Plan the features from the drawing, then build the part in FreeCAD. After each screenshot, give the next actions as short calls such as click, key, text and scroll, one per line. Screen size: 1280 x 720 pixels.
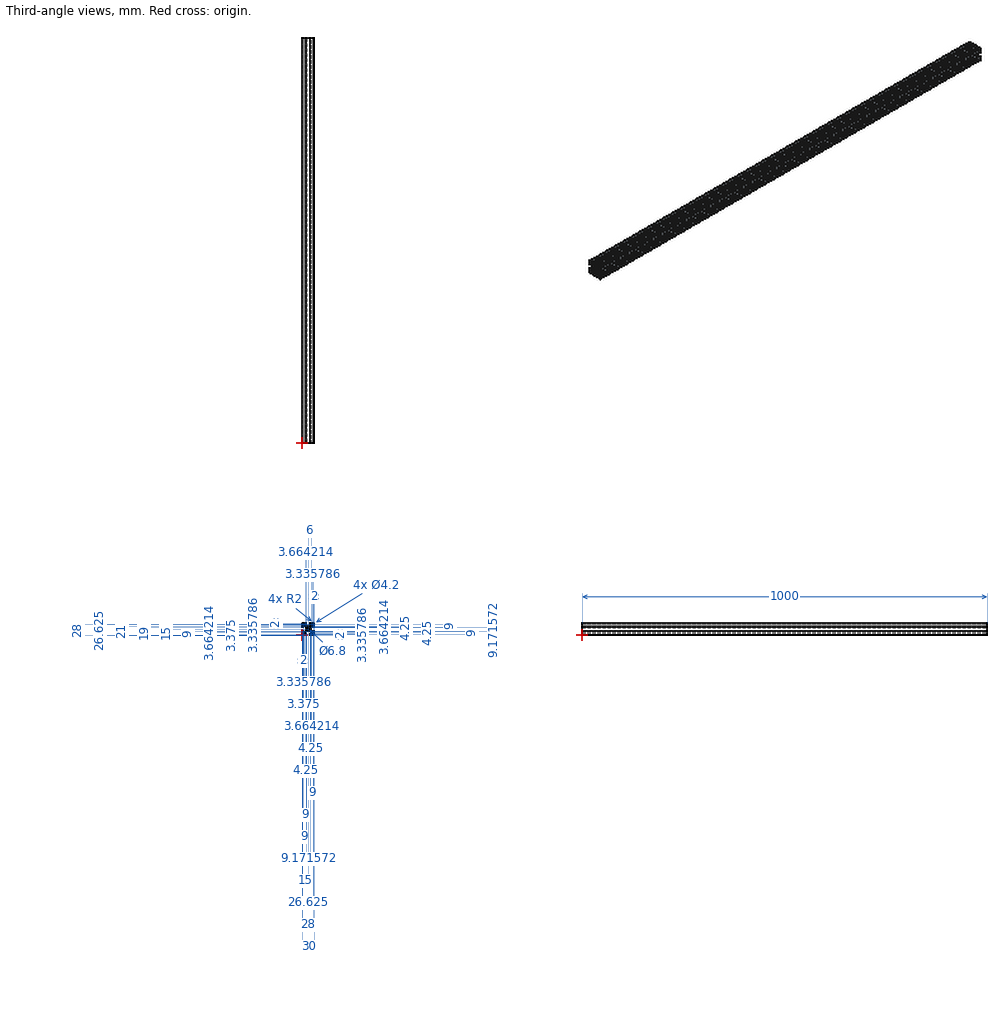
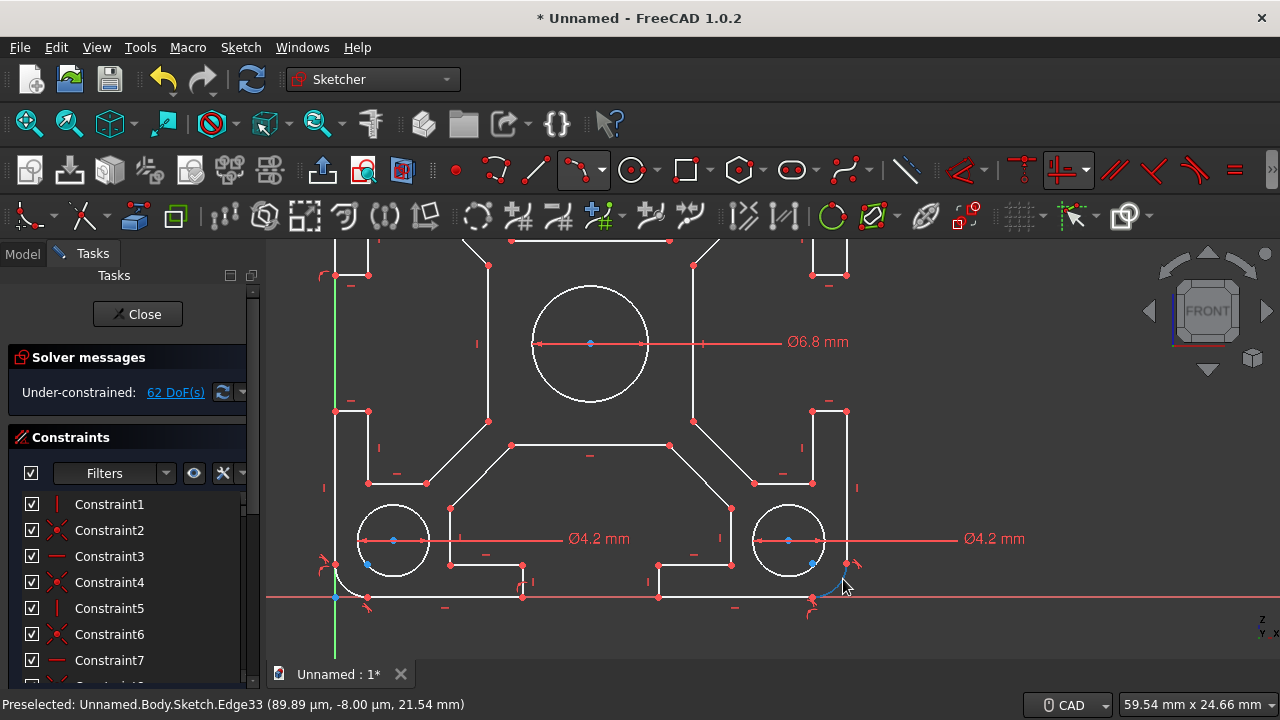
click(843, 579)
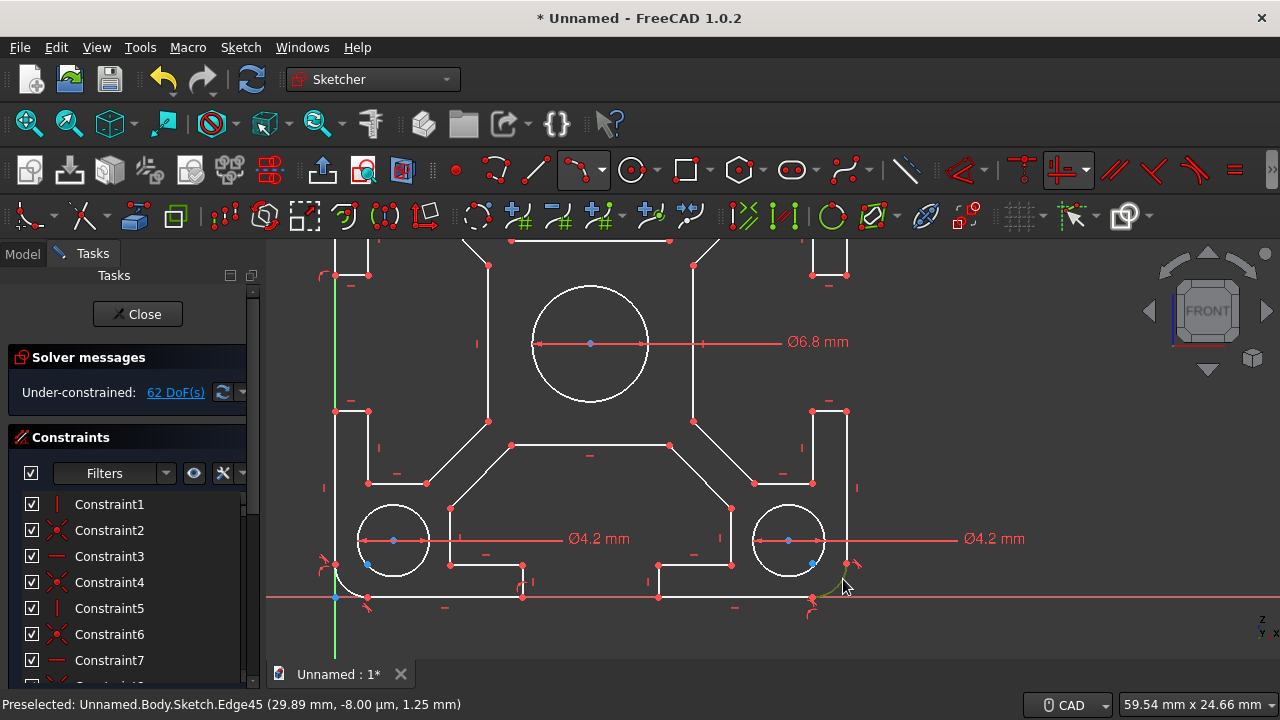
click(339, 579)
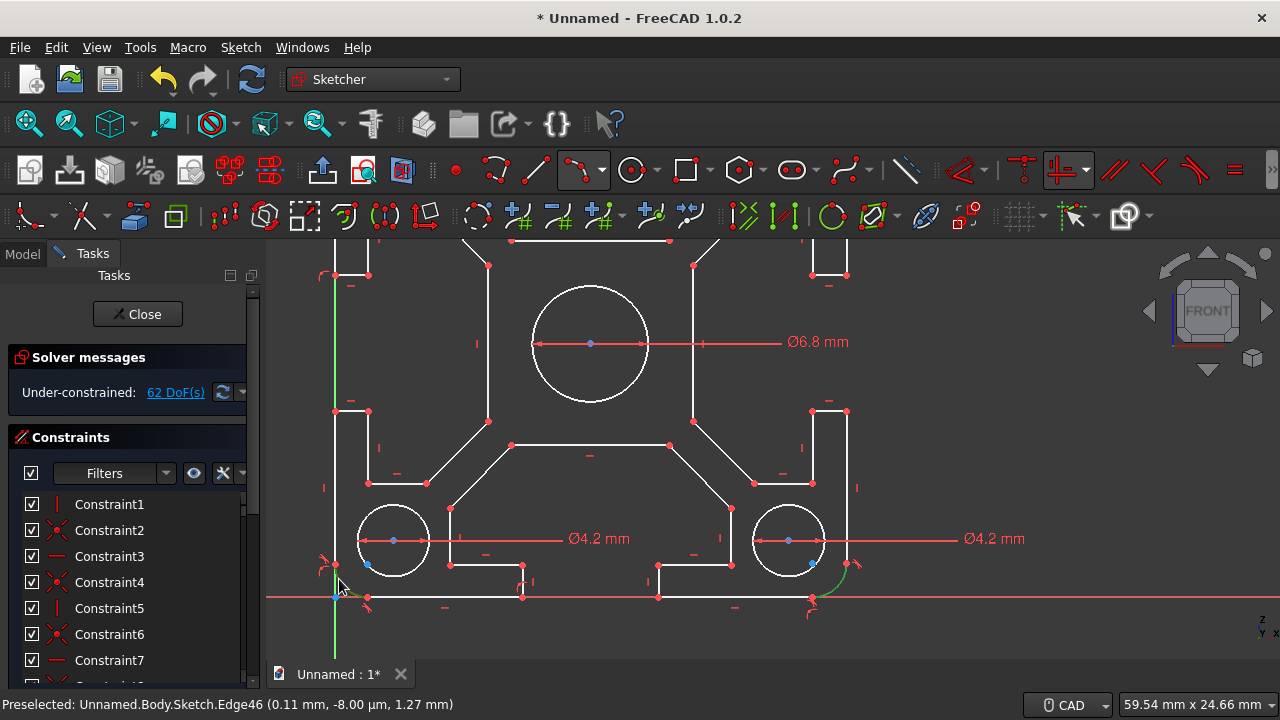
scroll(843, 580, down, 3)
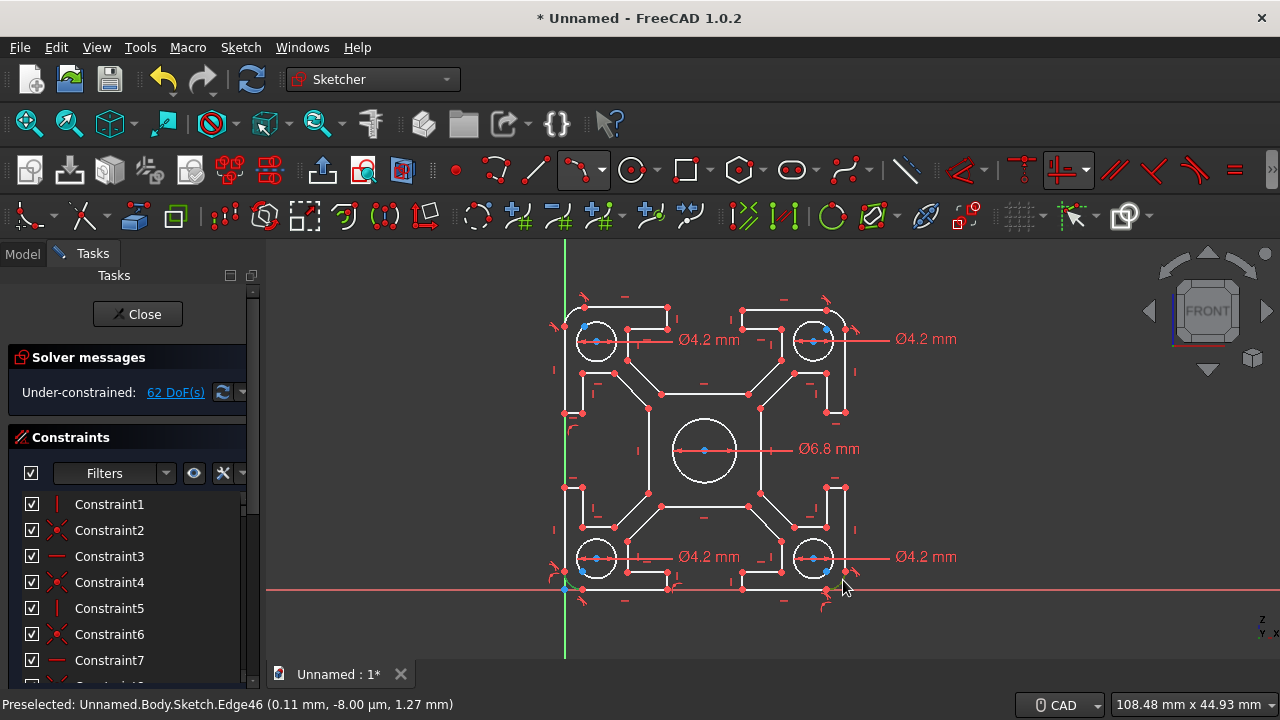
scroll(575, 309, up, 3)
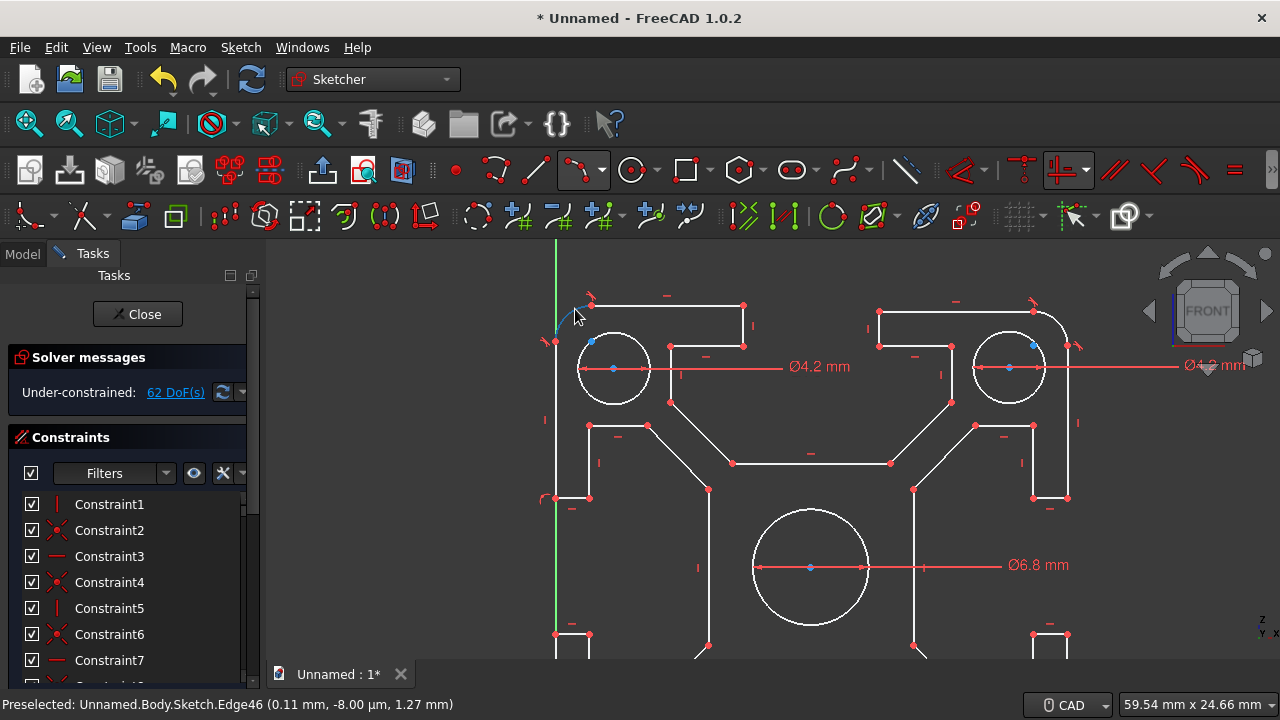
click(575, 310)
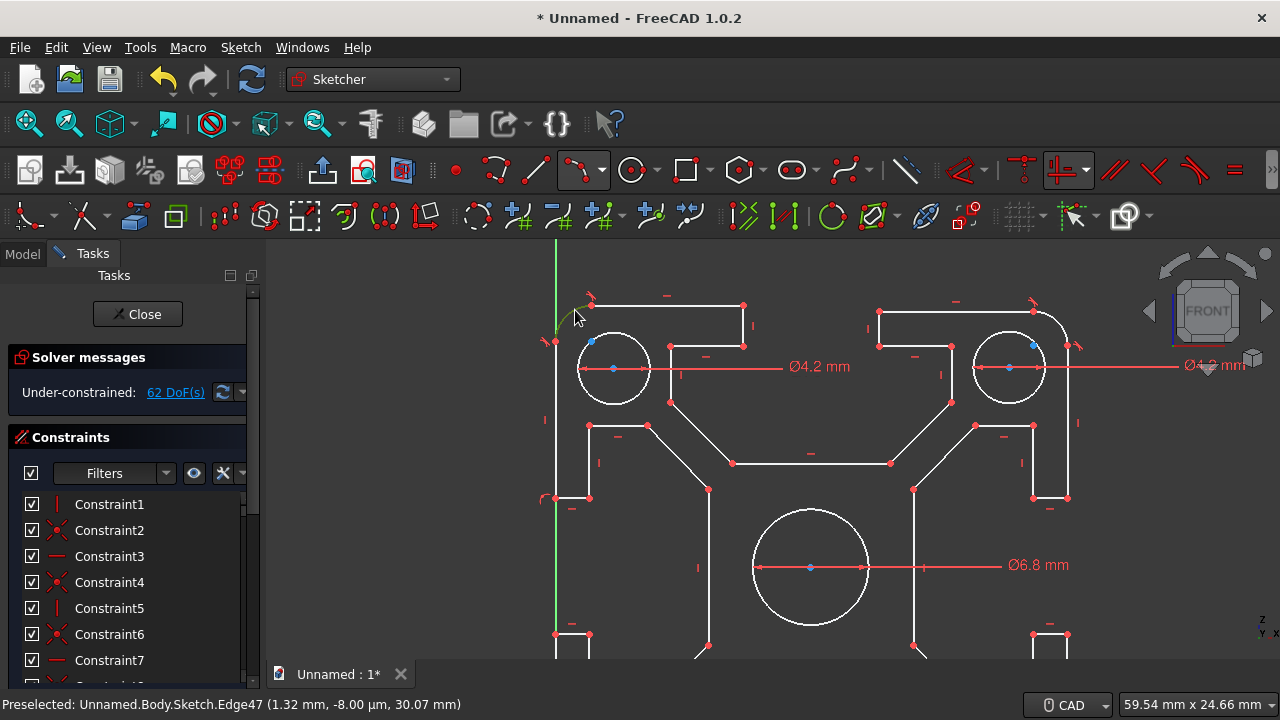
click(1064, 330)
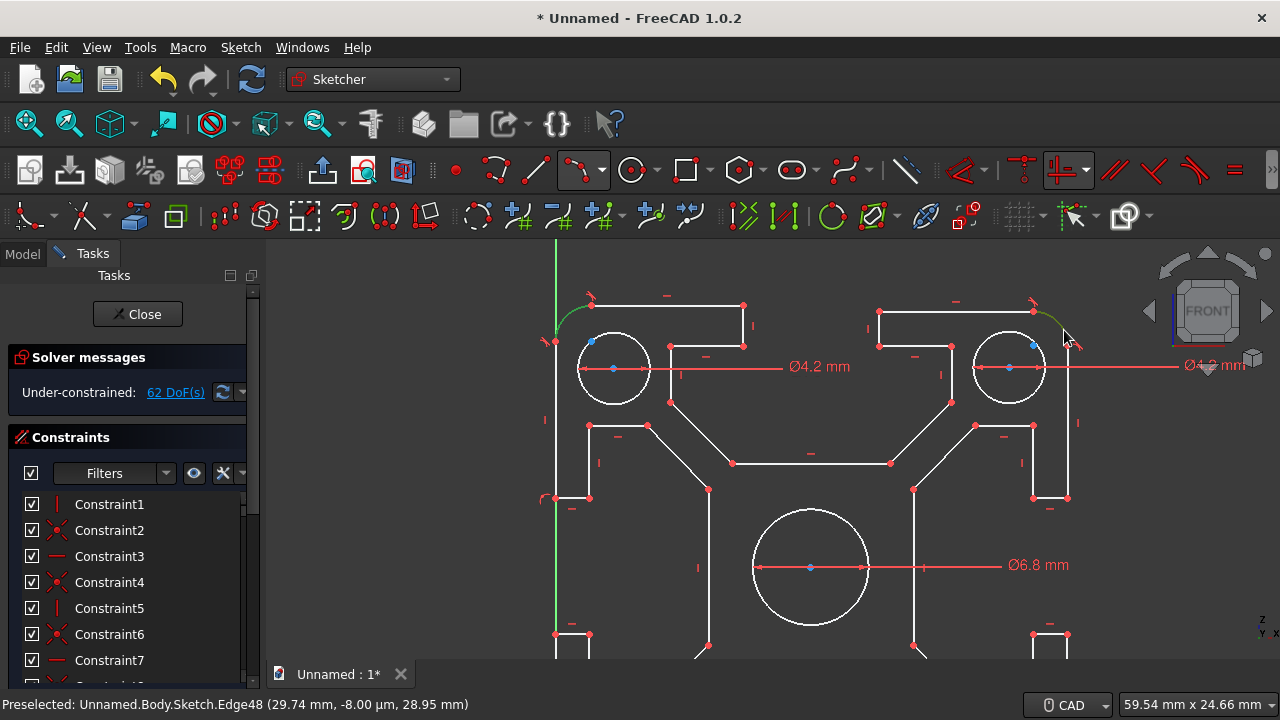
click(1236, 170)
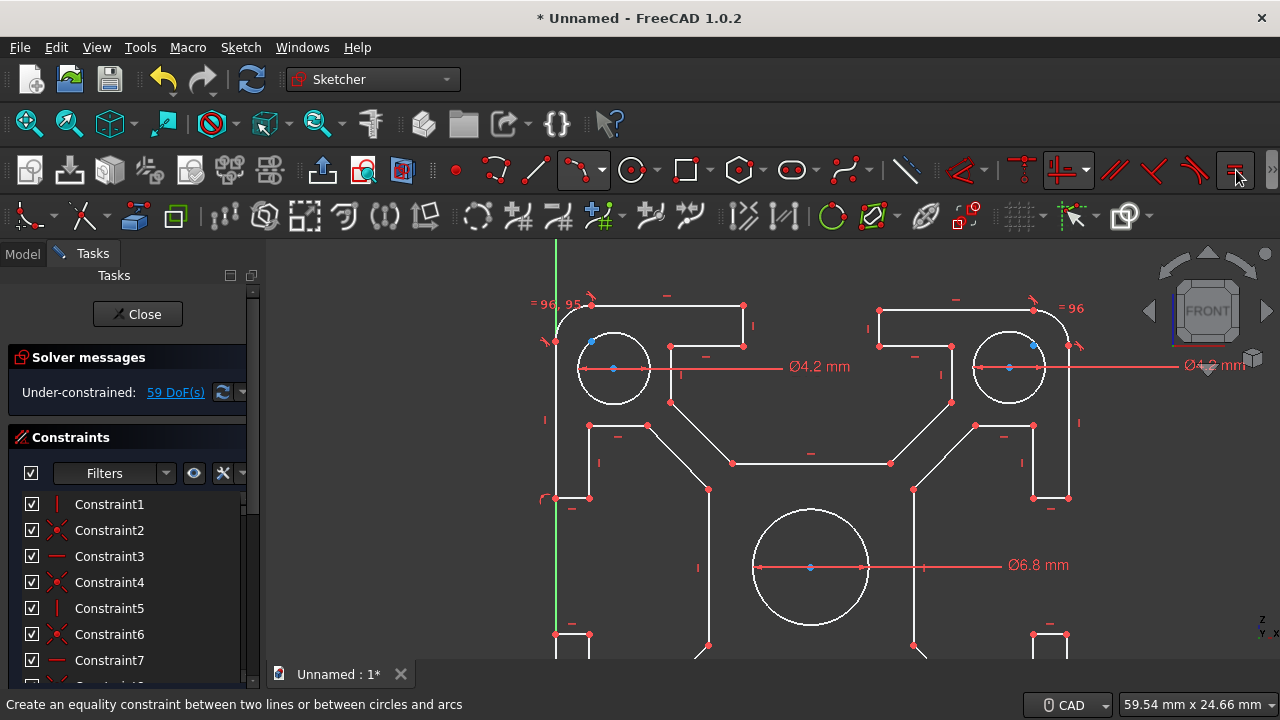
click(960, 170)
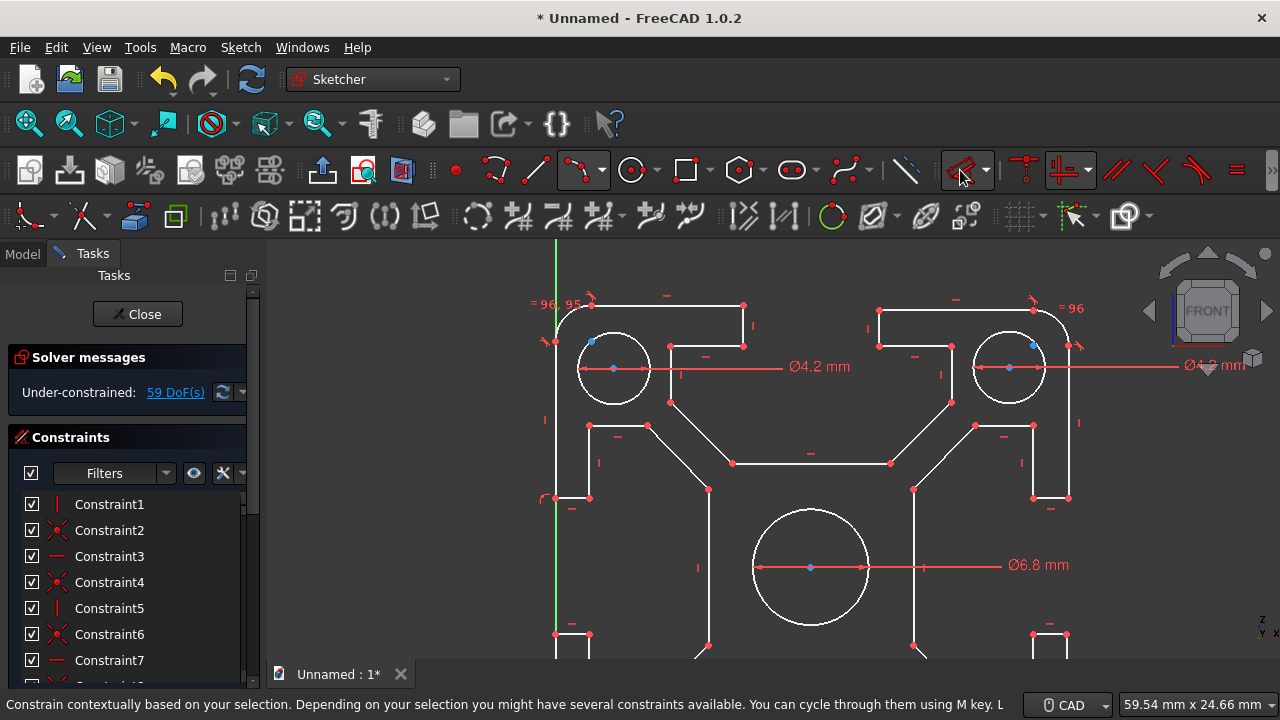
scroll(575, 308, down, 3)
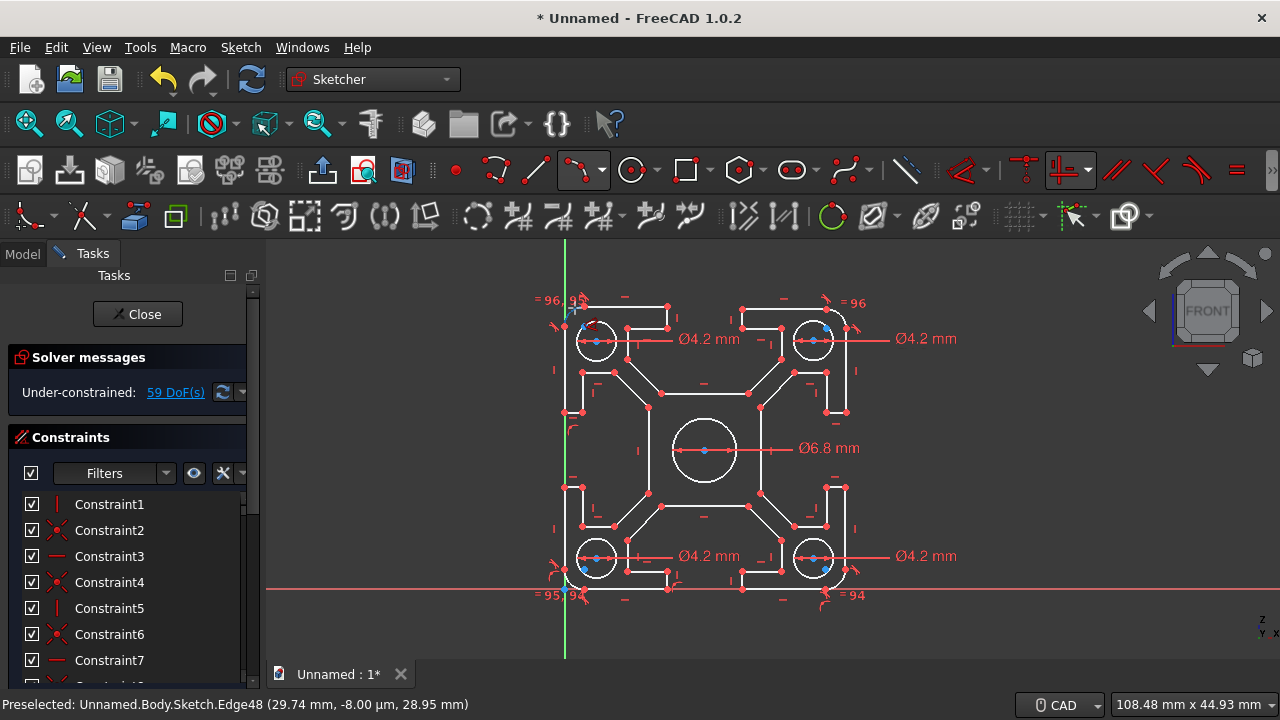
scroll(834, 587, up, 4)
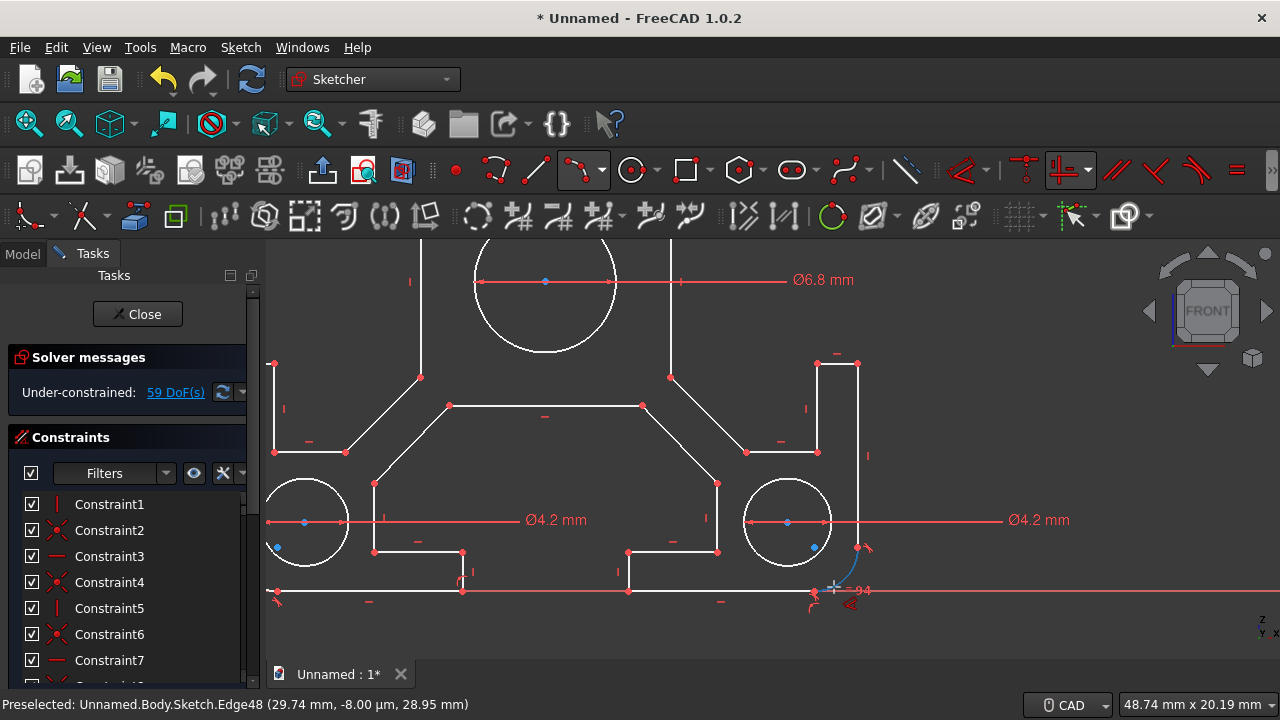
click(834, 586)
click(849, 615)